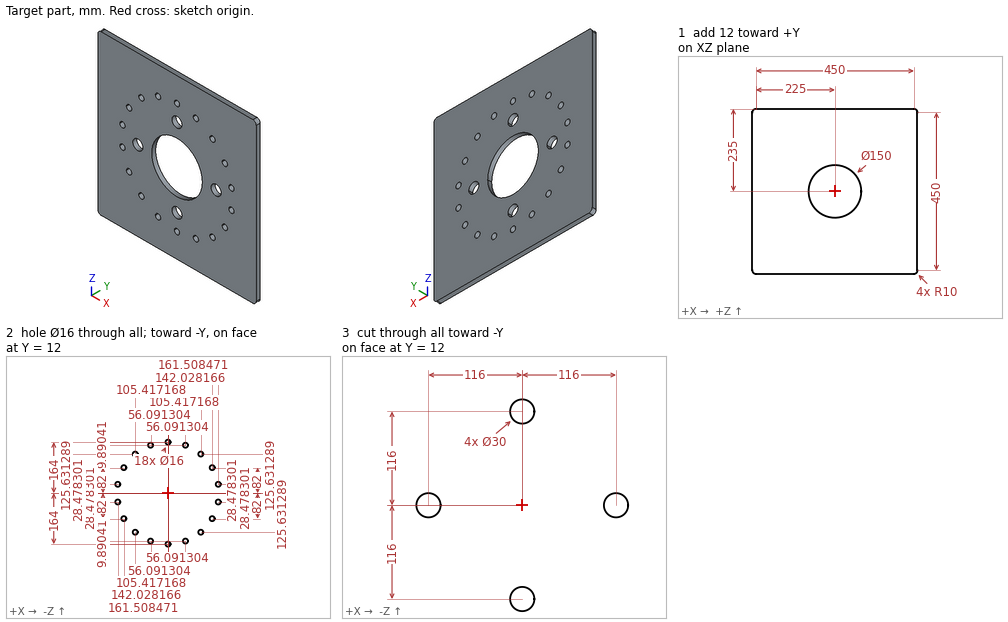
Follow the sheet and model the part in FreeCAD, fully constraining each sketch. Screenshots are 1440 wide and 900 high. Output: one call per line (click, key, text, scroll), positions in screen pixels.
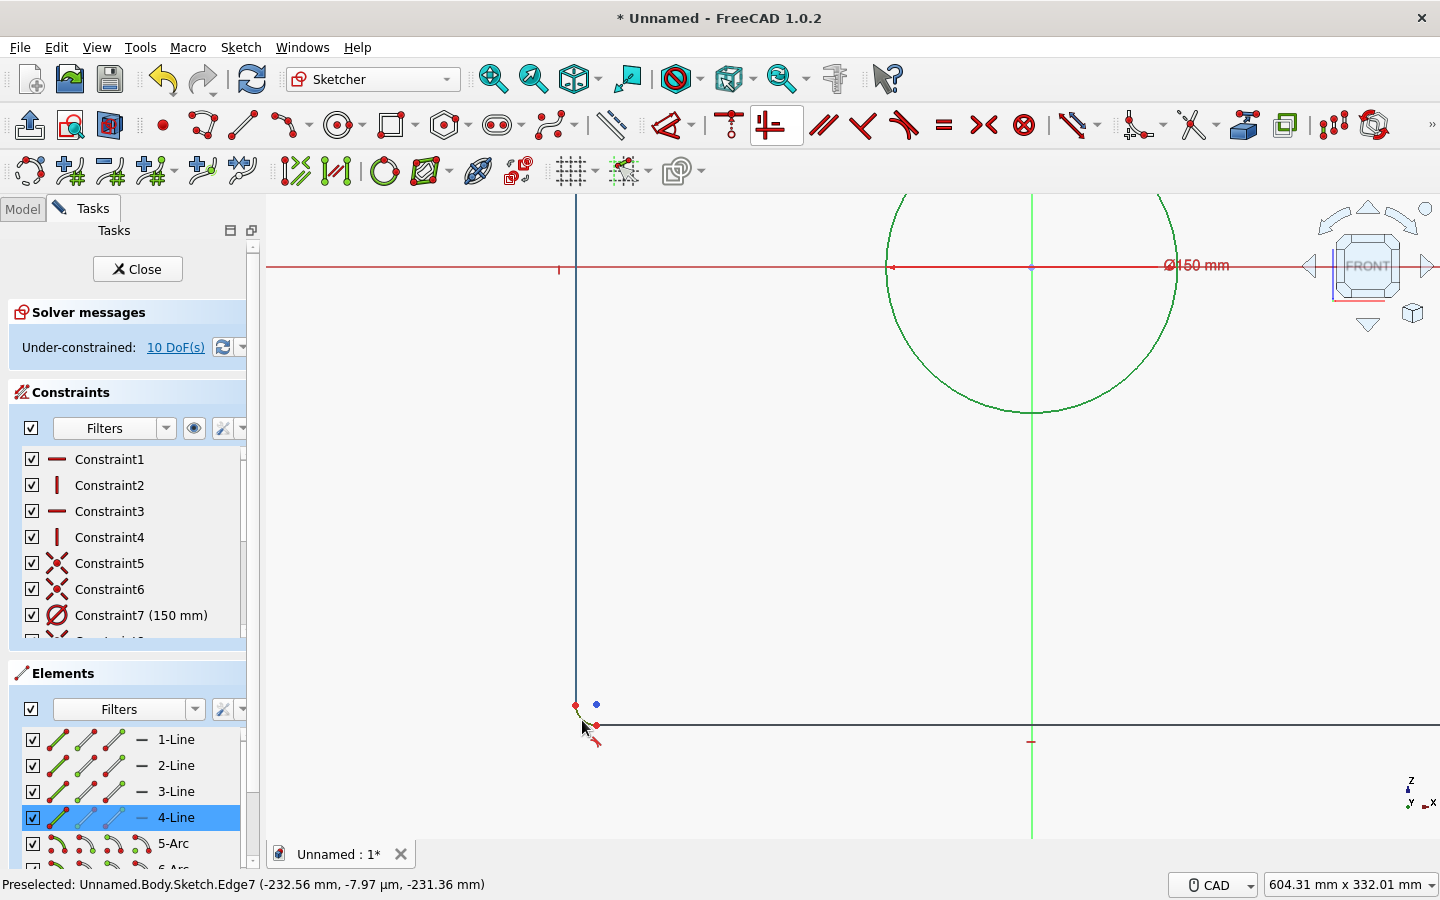
click(904, 126)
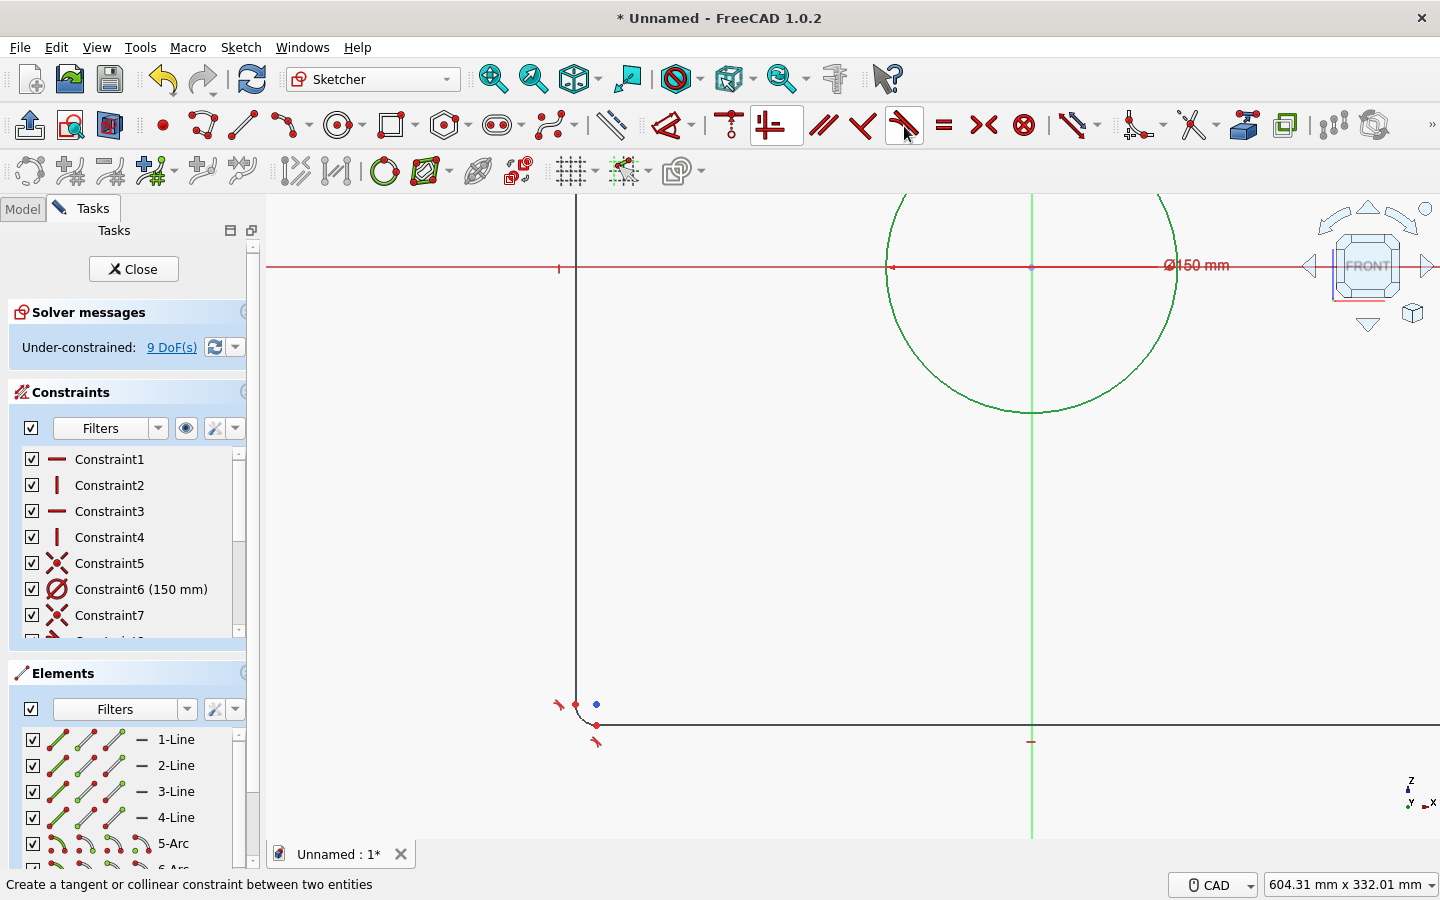
click(576, 443)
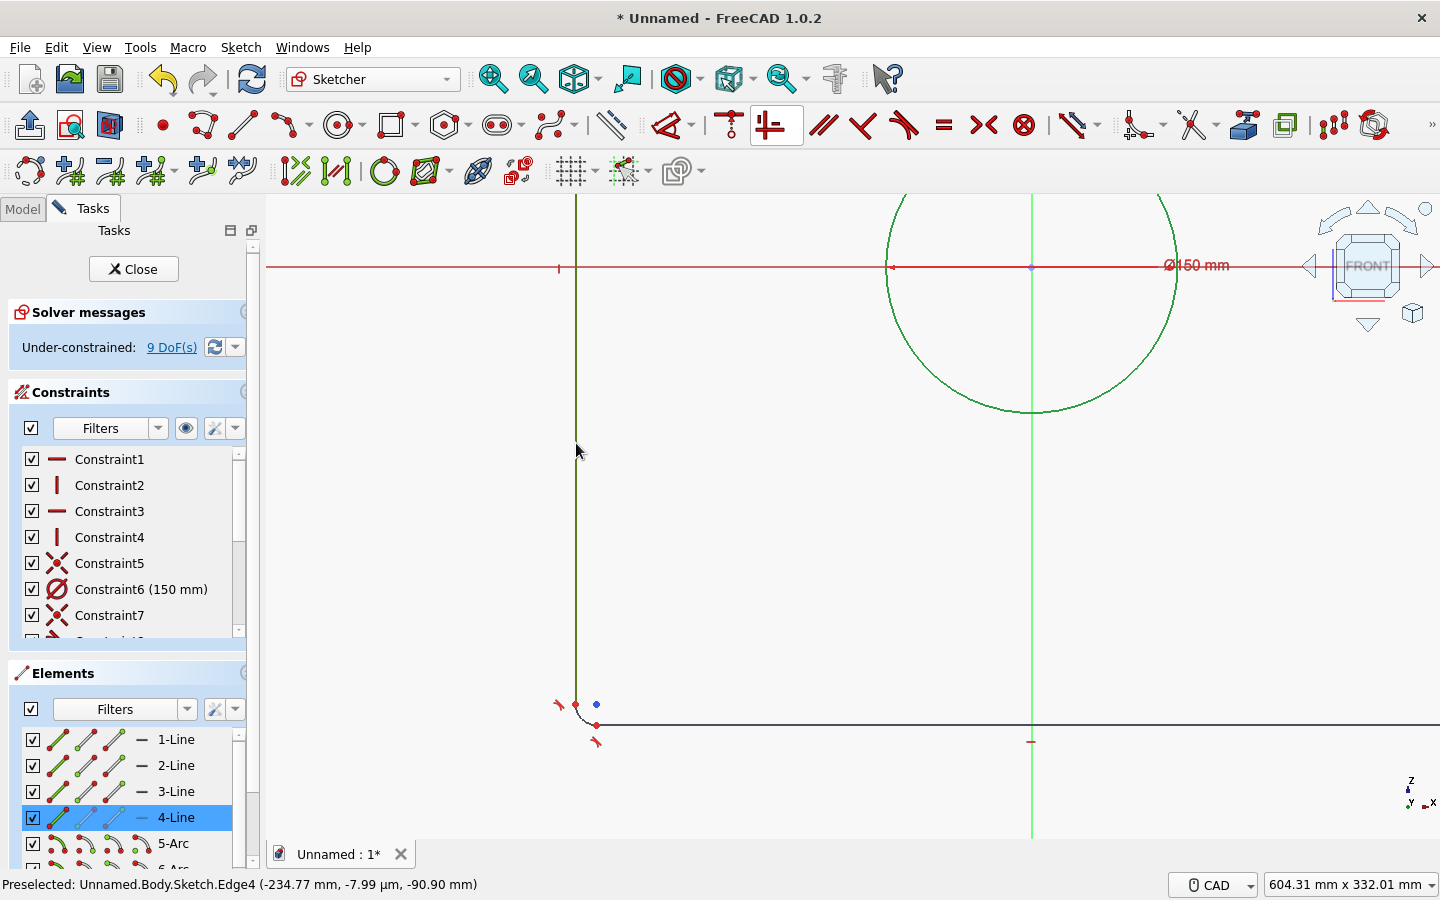
scroll(583, 720, down, 4)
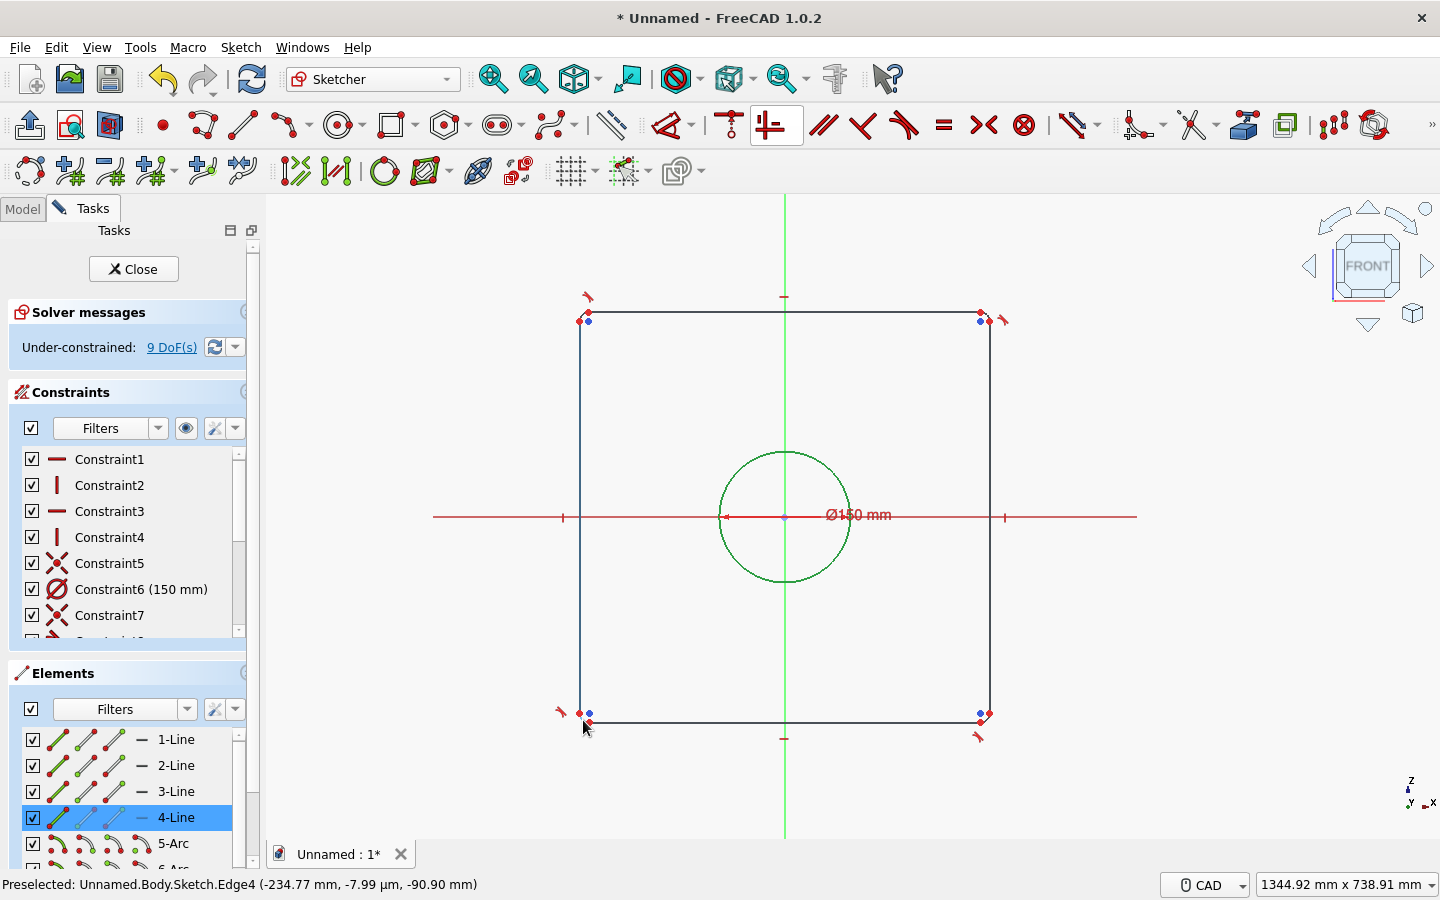
scroll(585, 313, up, 6)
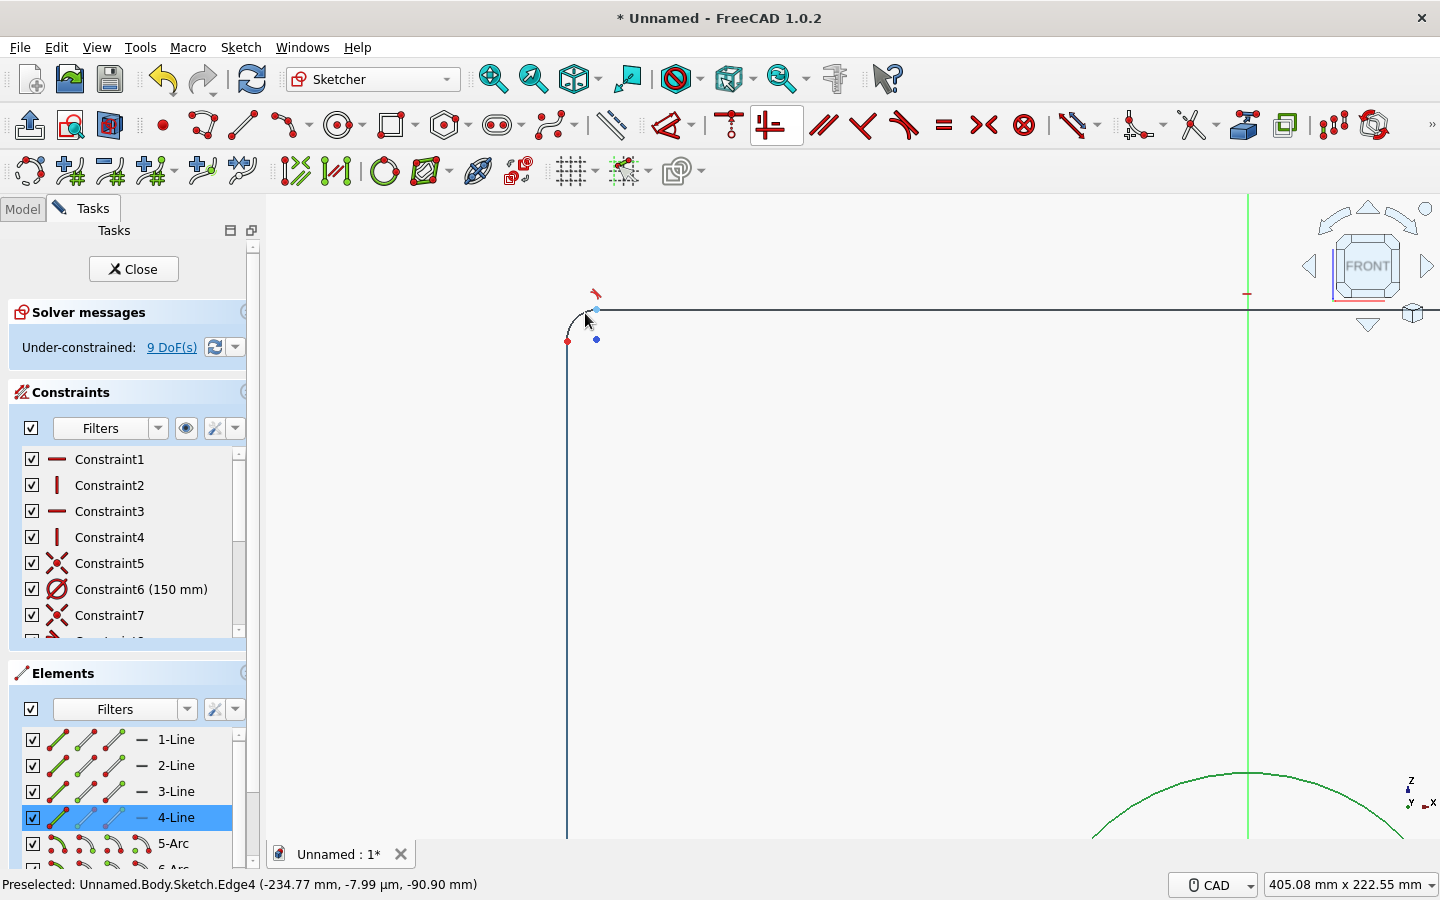
click(583, 313)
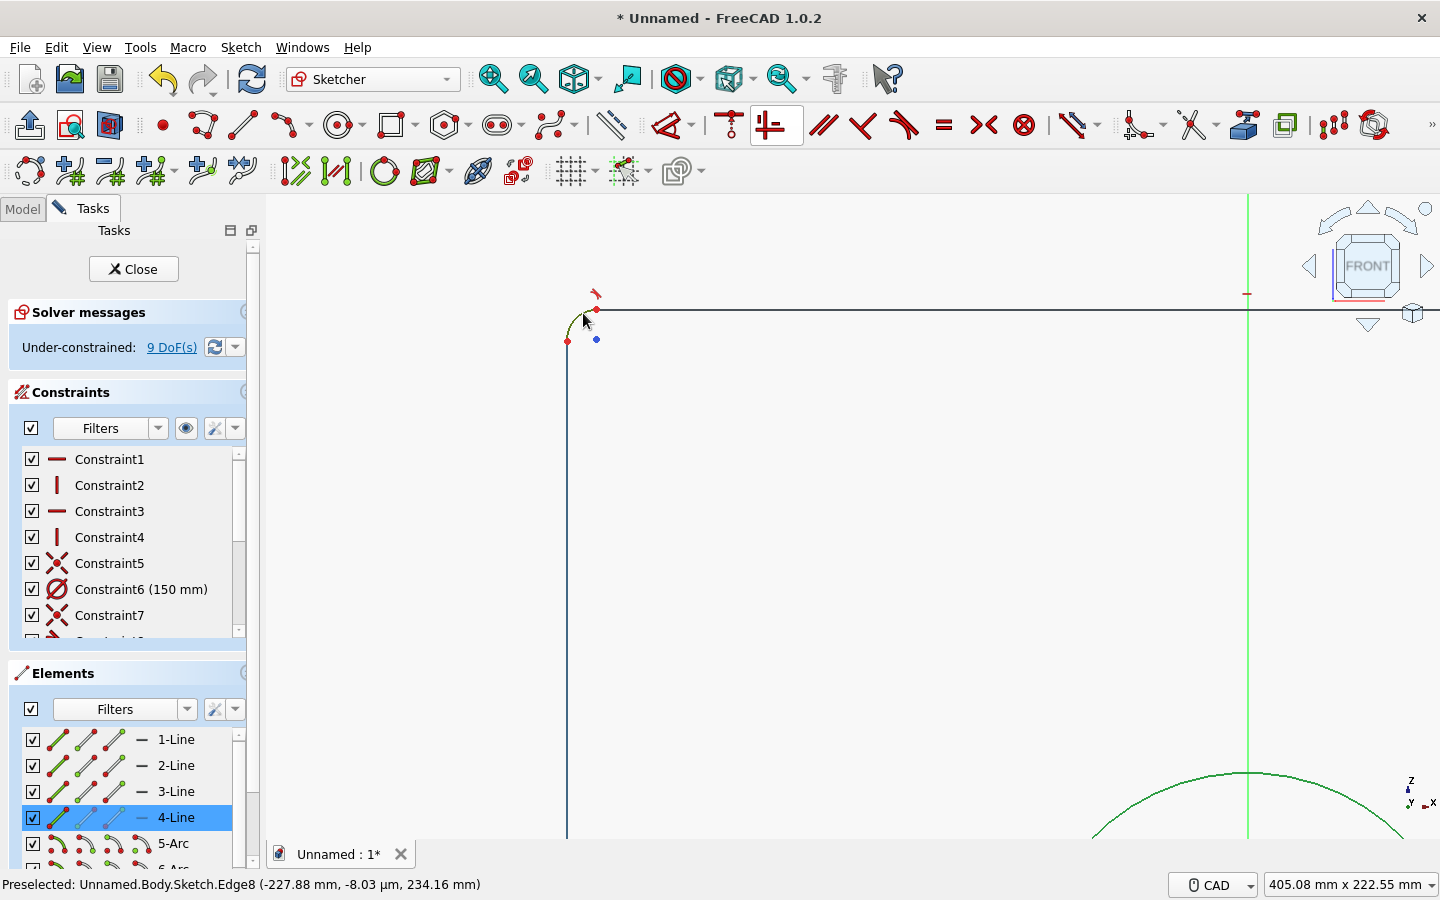
click(904, 126)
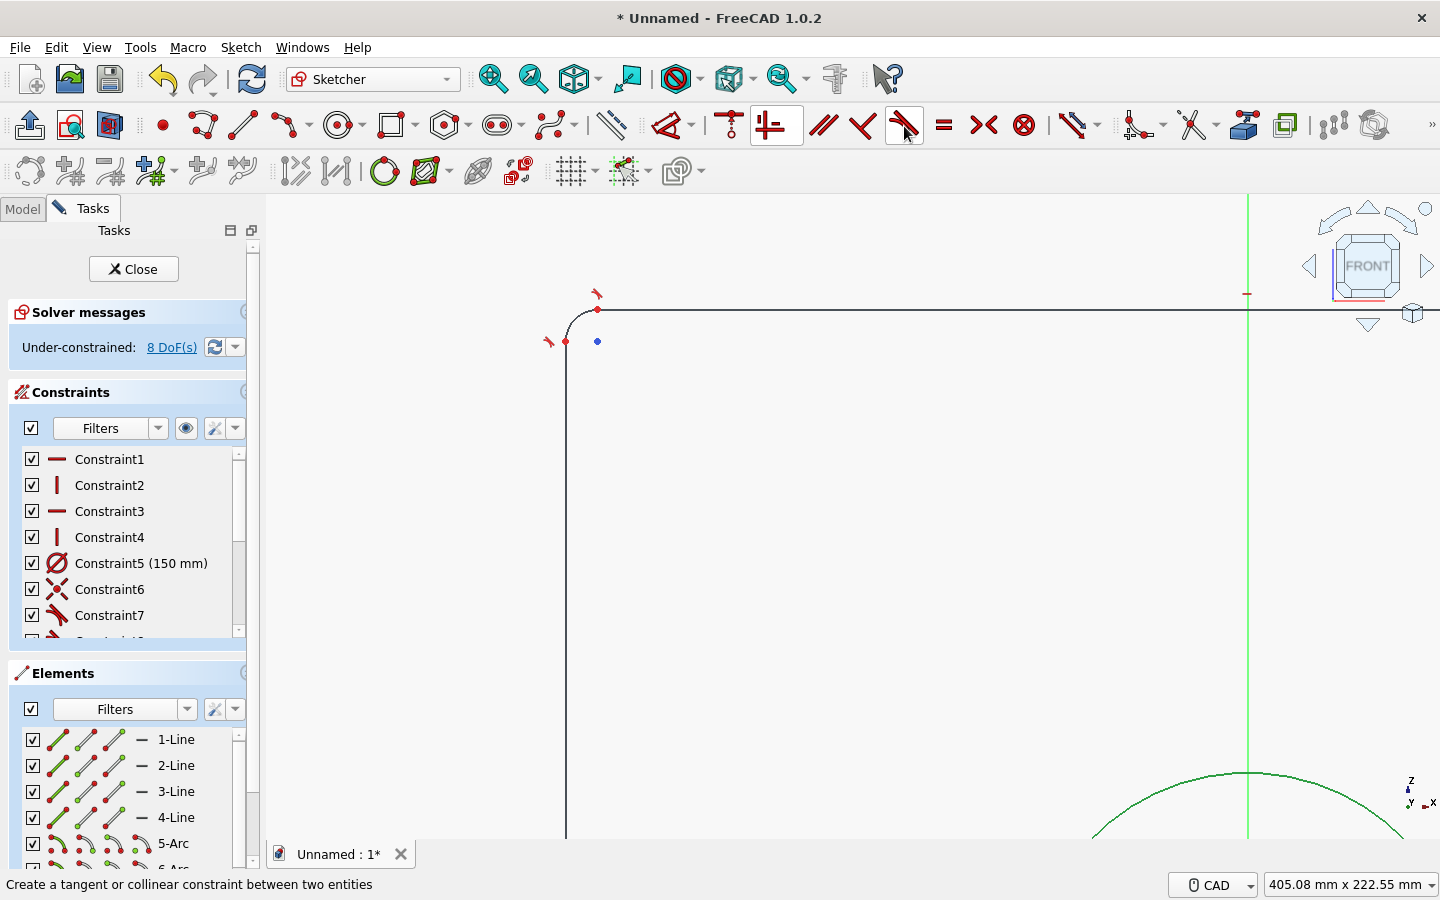
scroll(585, 312, down, 6)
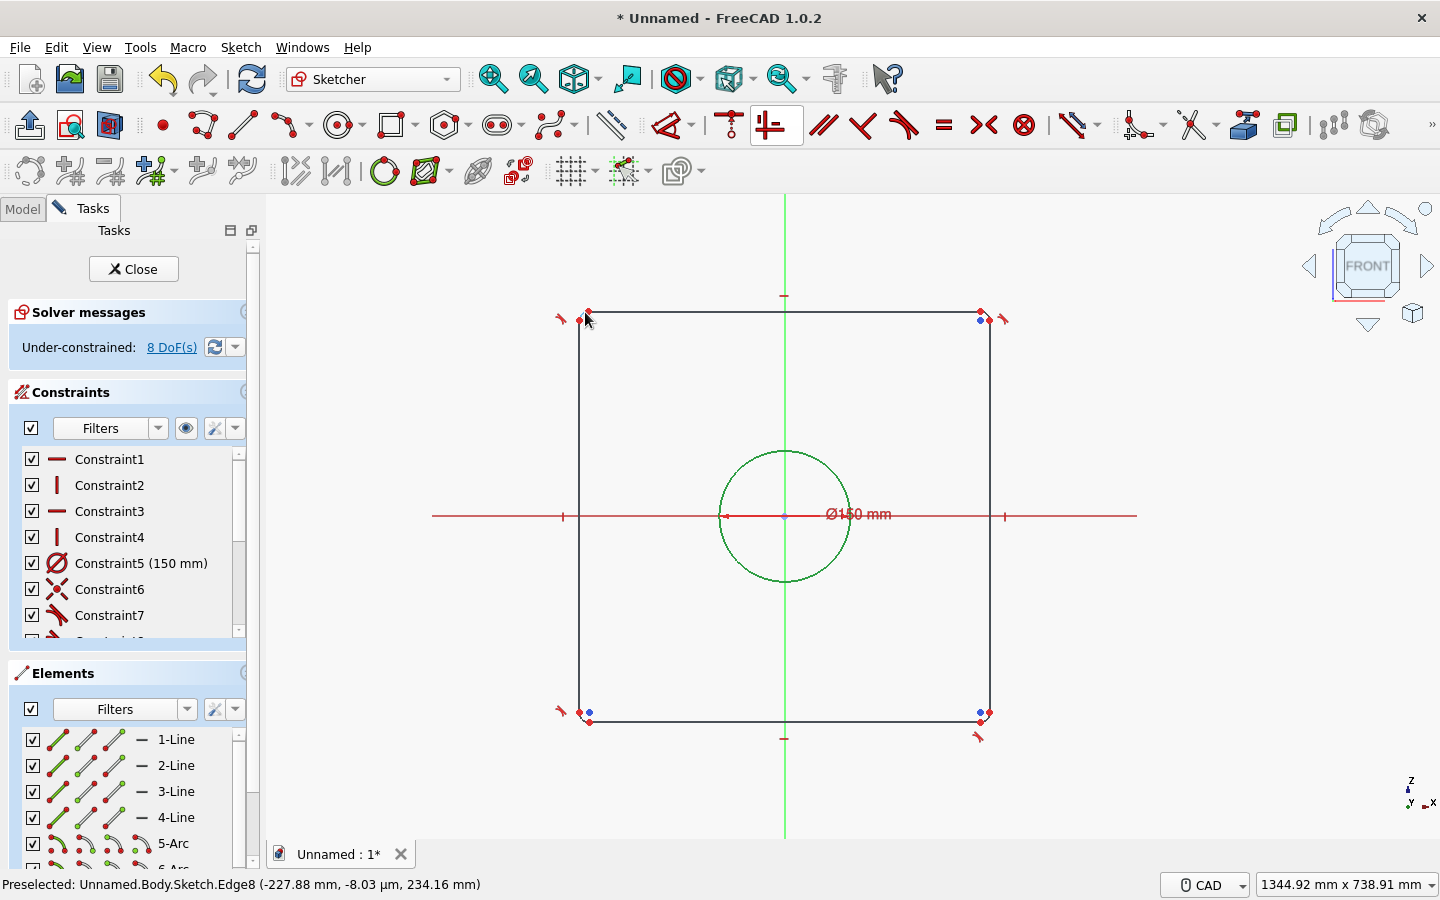
scroll(989, 317, up, 6)